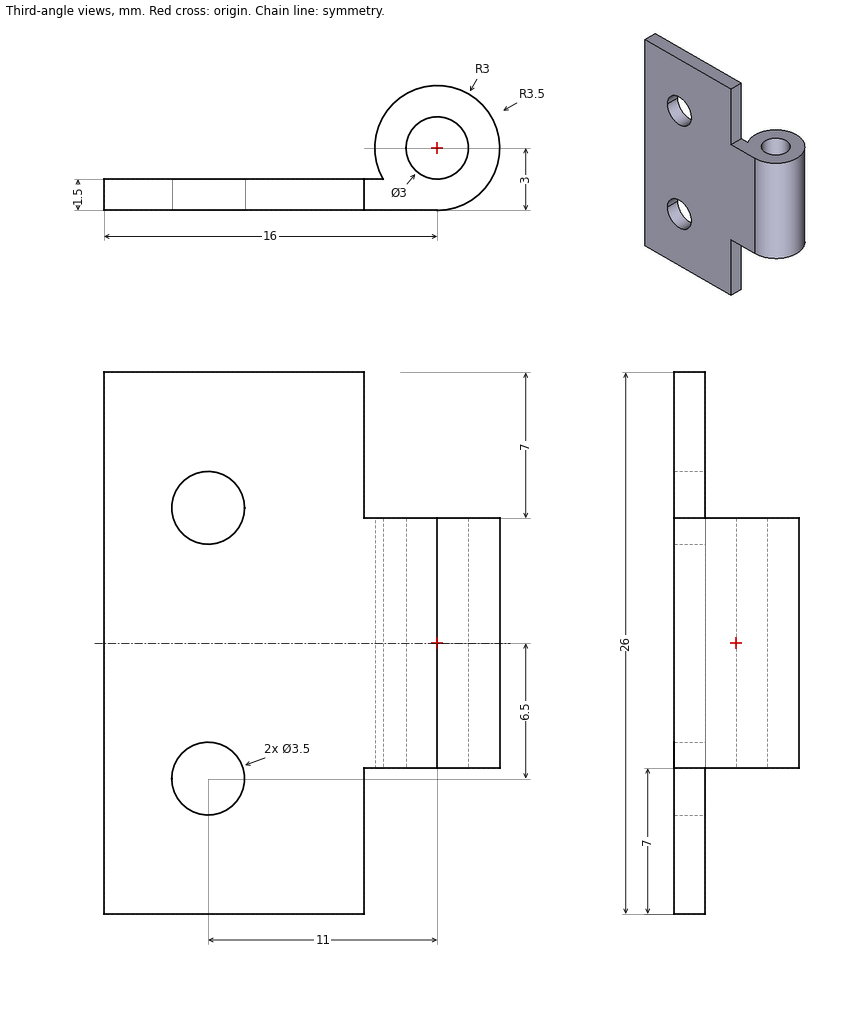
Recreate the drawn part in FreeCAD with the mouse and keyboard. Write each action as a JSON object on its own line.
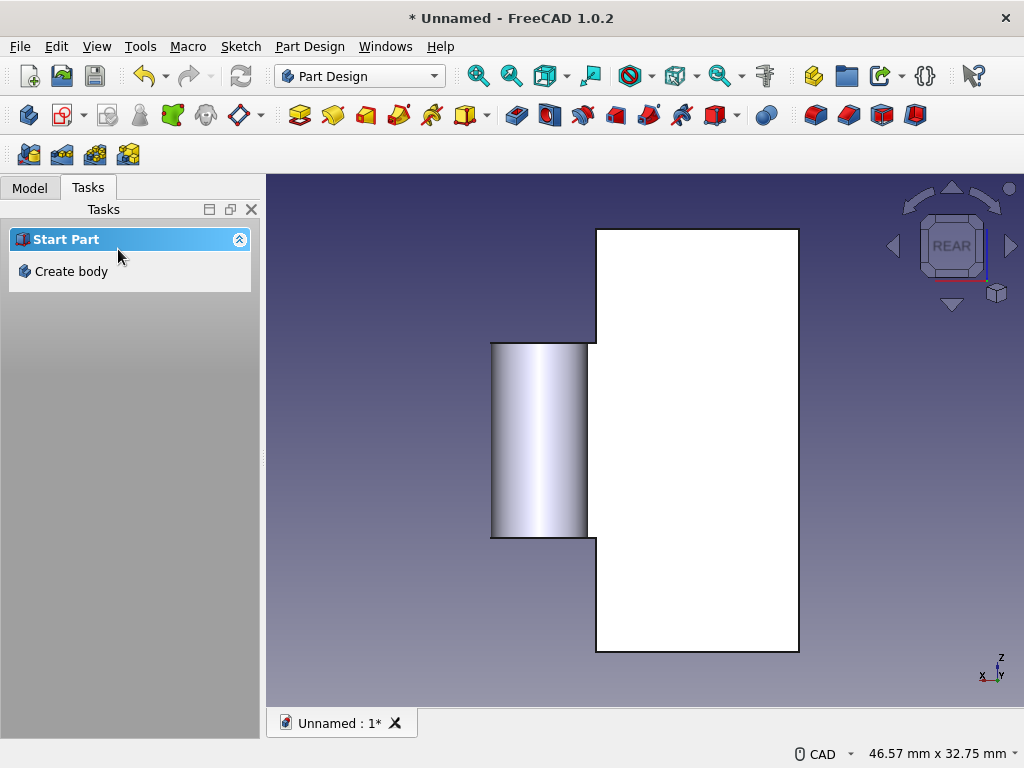
{"action": "left_click", "coordinate": [690, 439]}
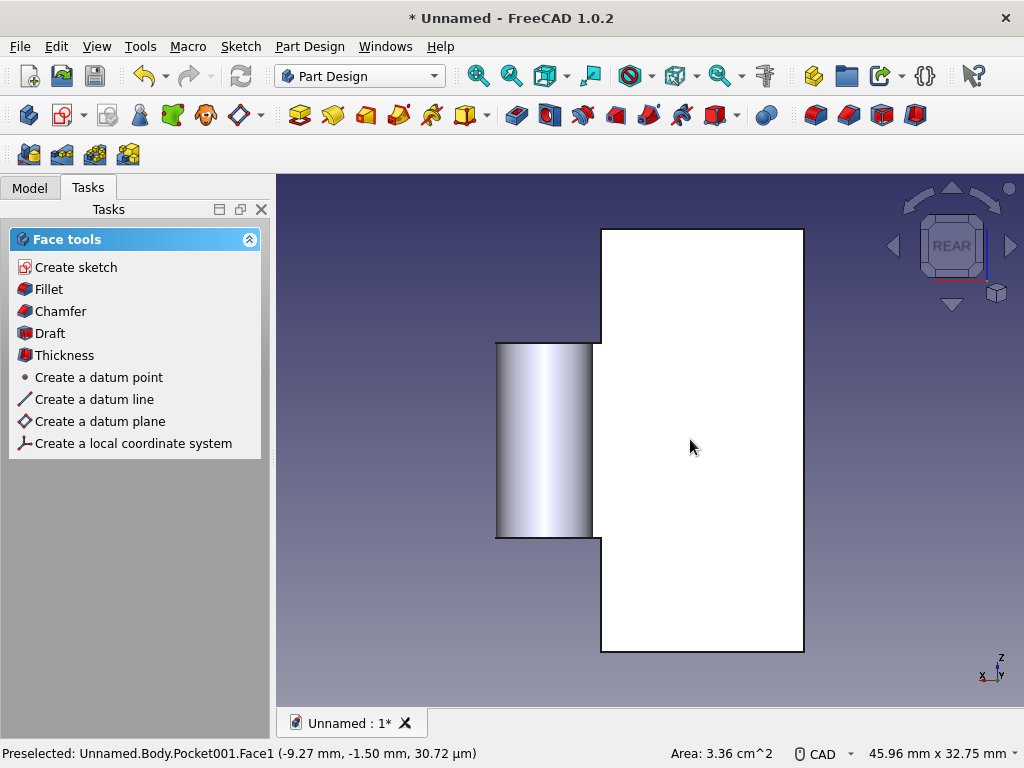
{"action": "left_click", "coordinate": [62, 116]}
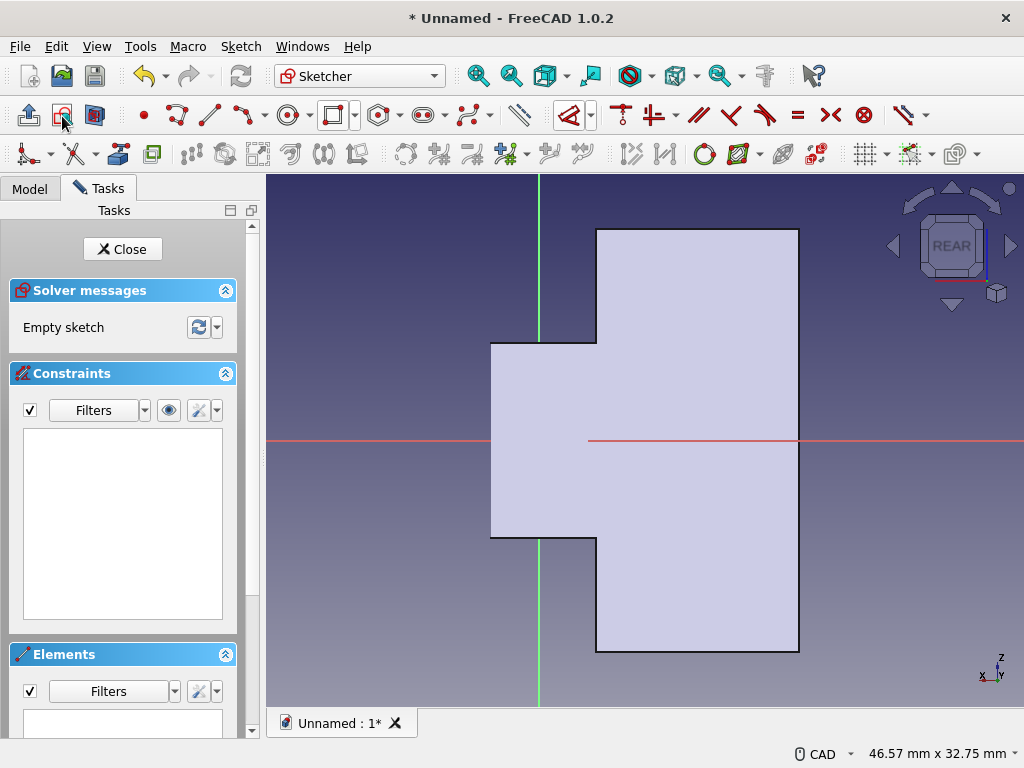
{"action": "left_click", "coordinate": [288, 116]}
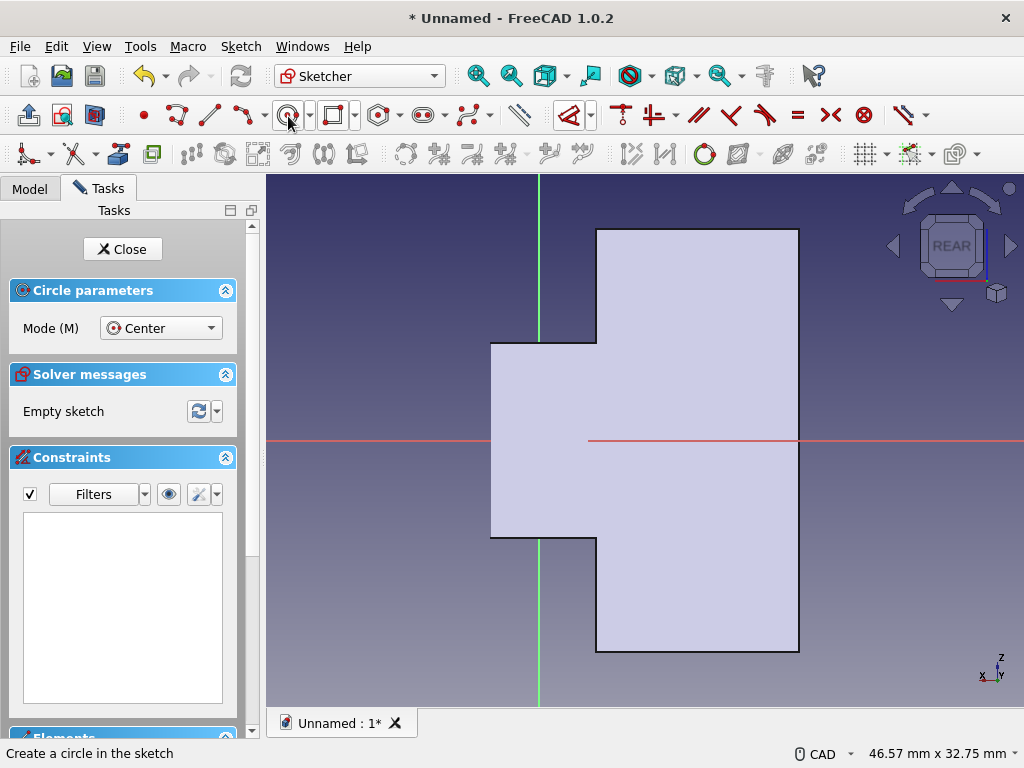
{"action": "left_click", "coordinate": [718, 546]}
{"action": "left_click", "coordinate": [738, 526]}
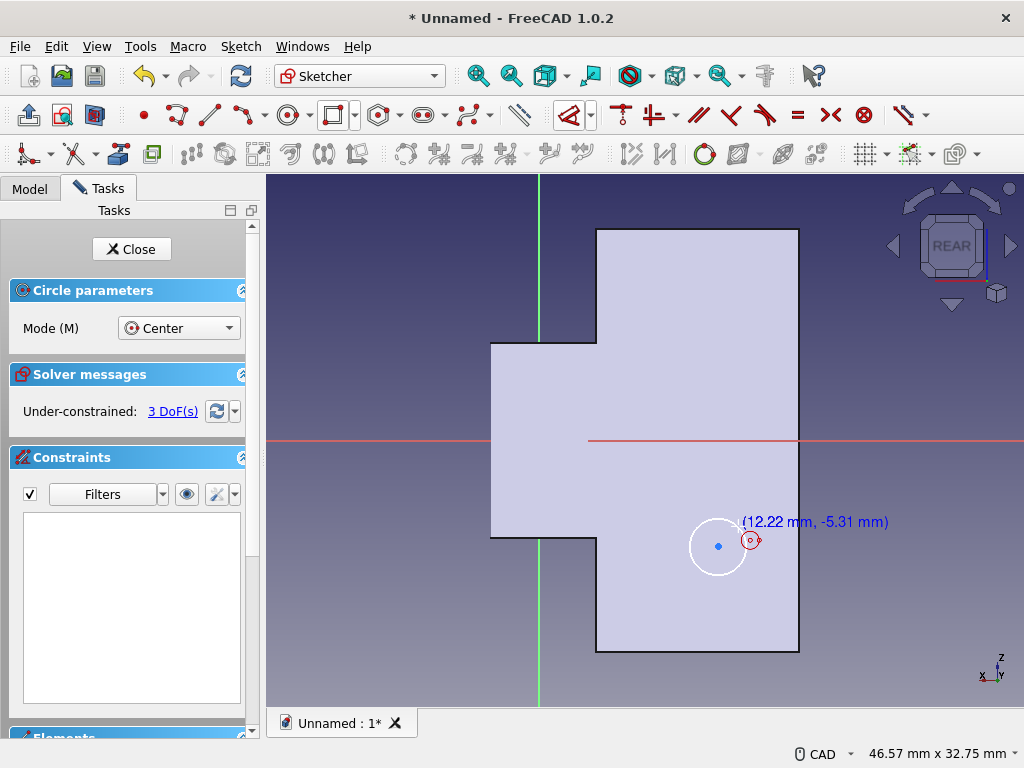
{"action": "left_click", "coordinate": [718, 335]}
{"action": "left_click", "coordinate": [738, 315]}
{"action": "key", "text": "Escape"}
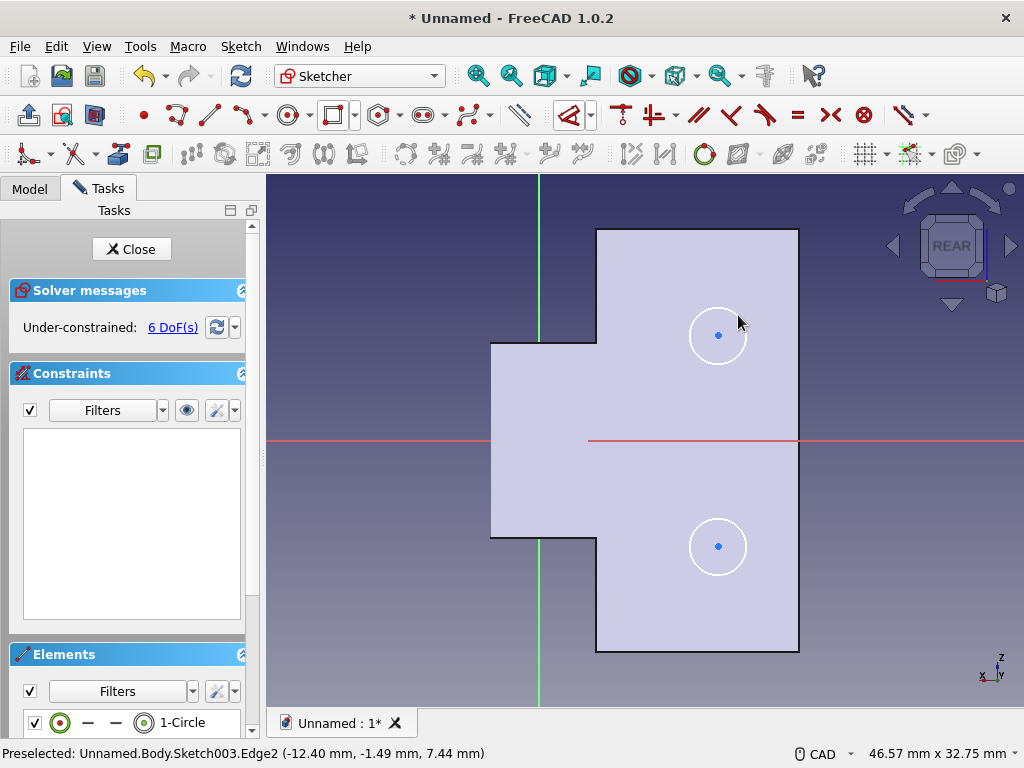
{"action": "left_click", "coordinate": [738, 527]}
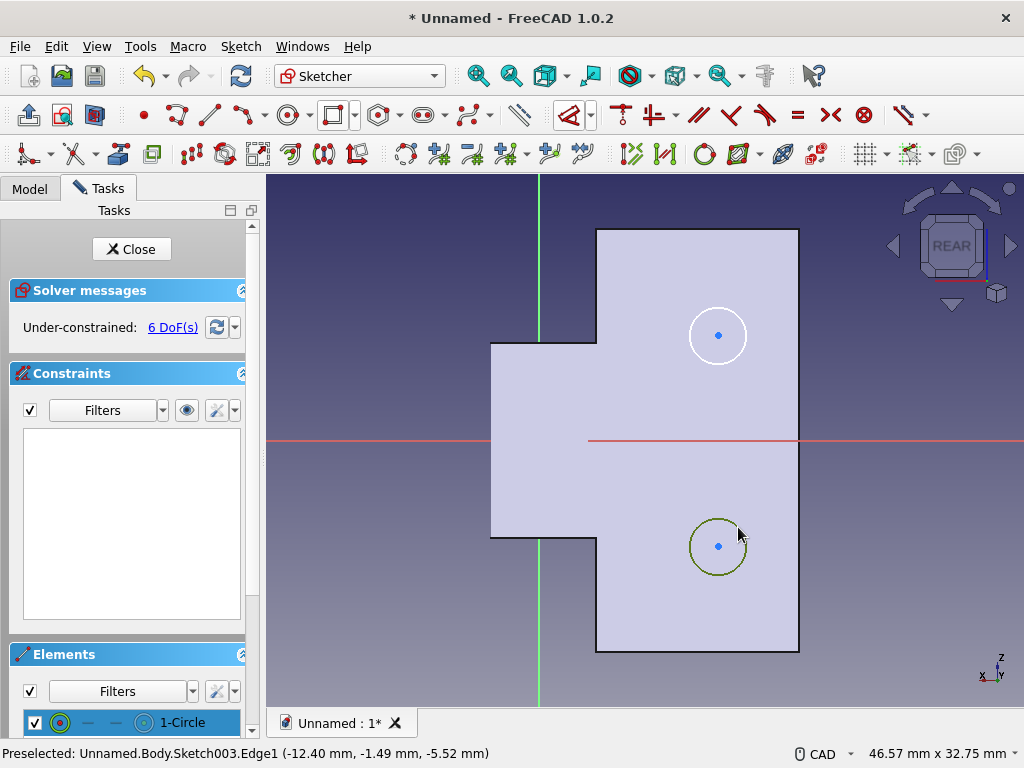
{"action": "left_click", "coordinate": [738, 316]}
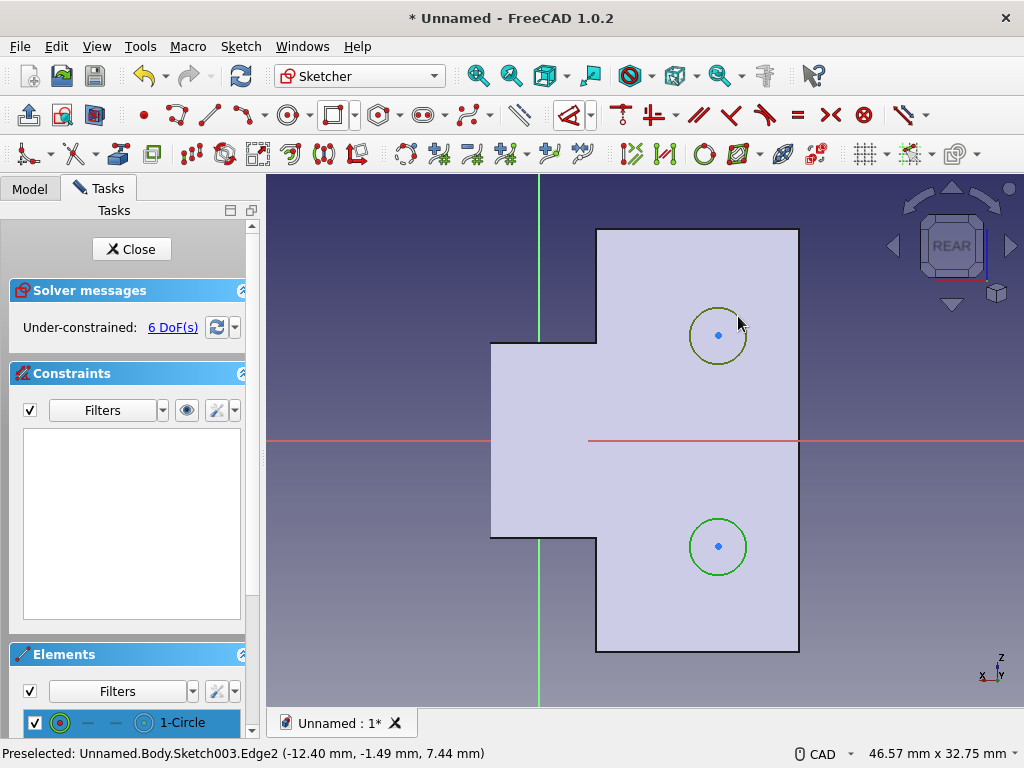
{"action": "left_click", "coordinate": [798, 116]}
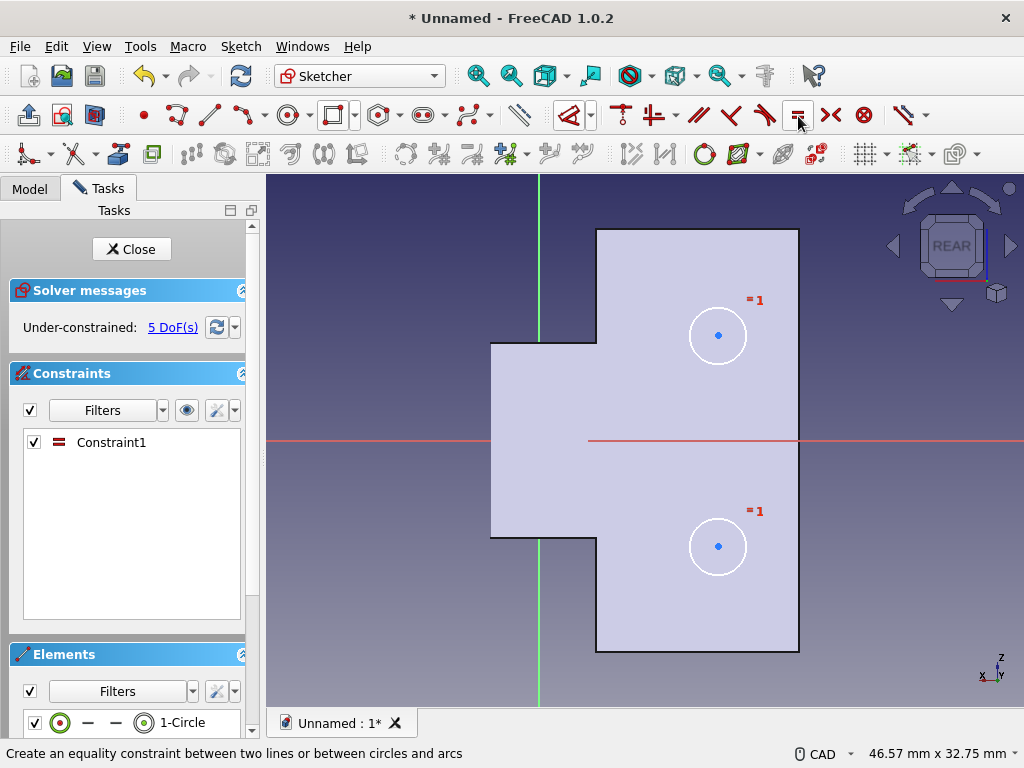
{"action": "left_click", "coordinate": [718, 547]}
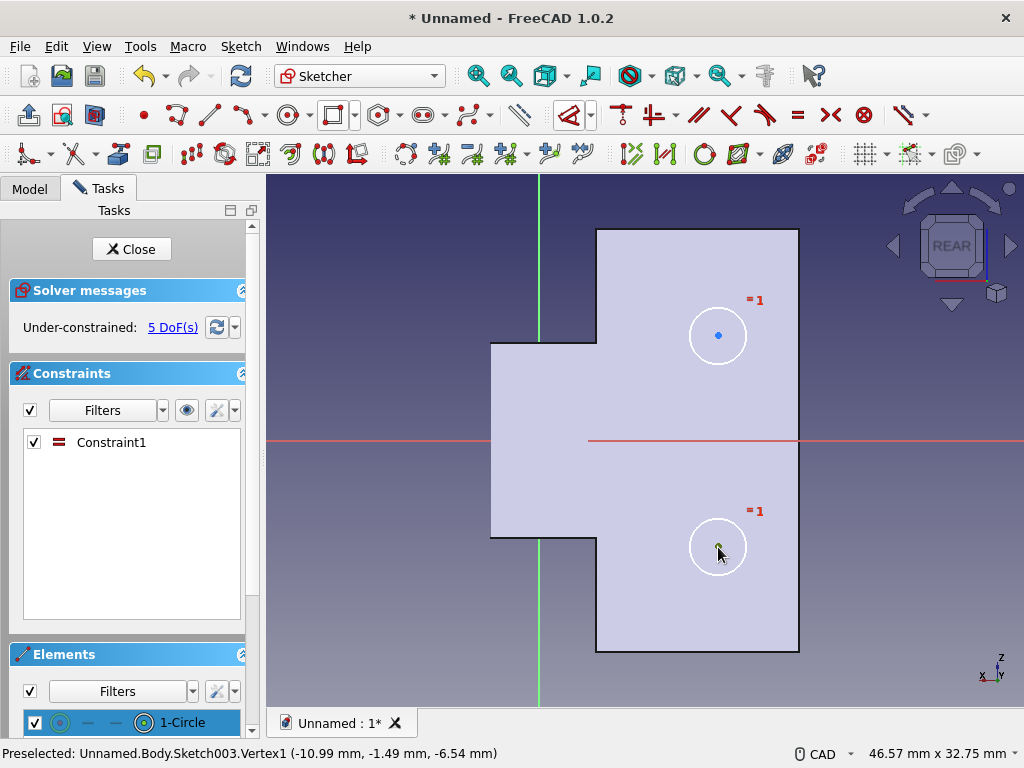
{"action": "left_click", "coordinate": [718, 336]}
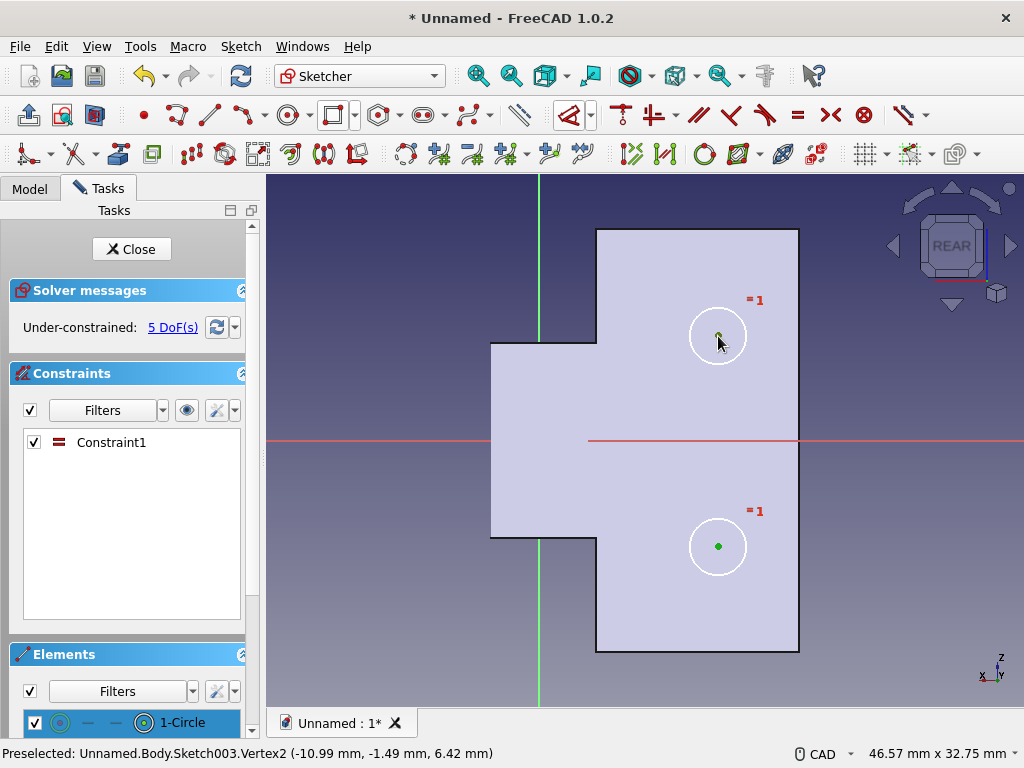
{"action": "left_click", "coordinate": [334, 440]}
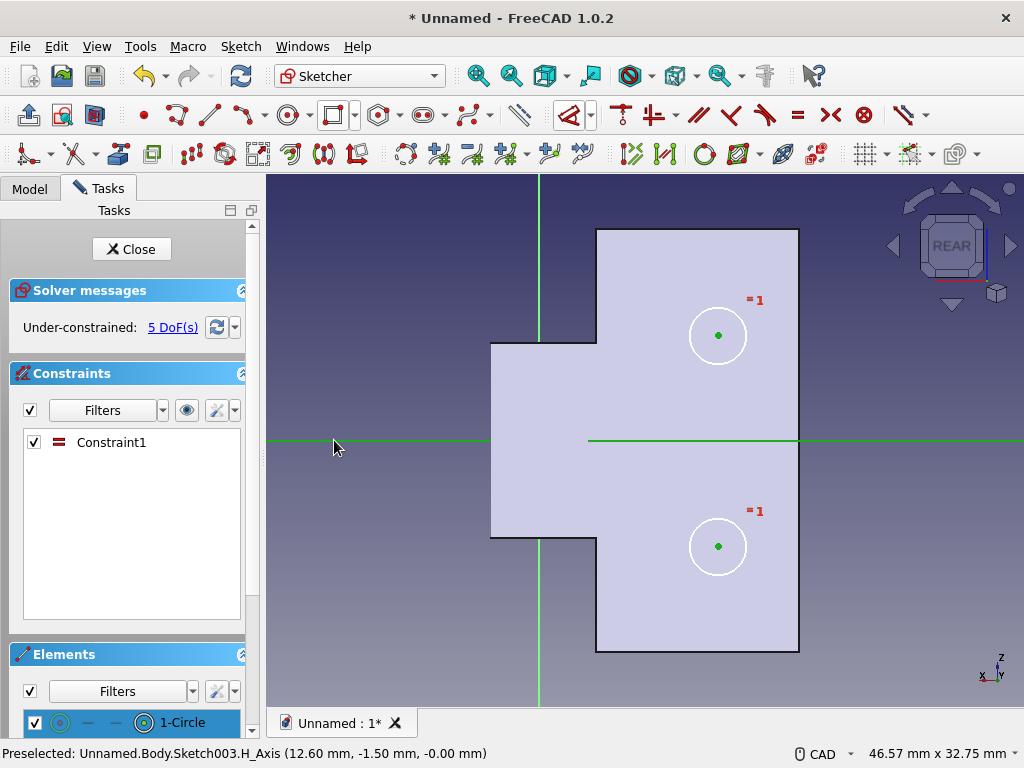
{"action": "left_click", "coordinate": [831, 116]}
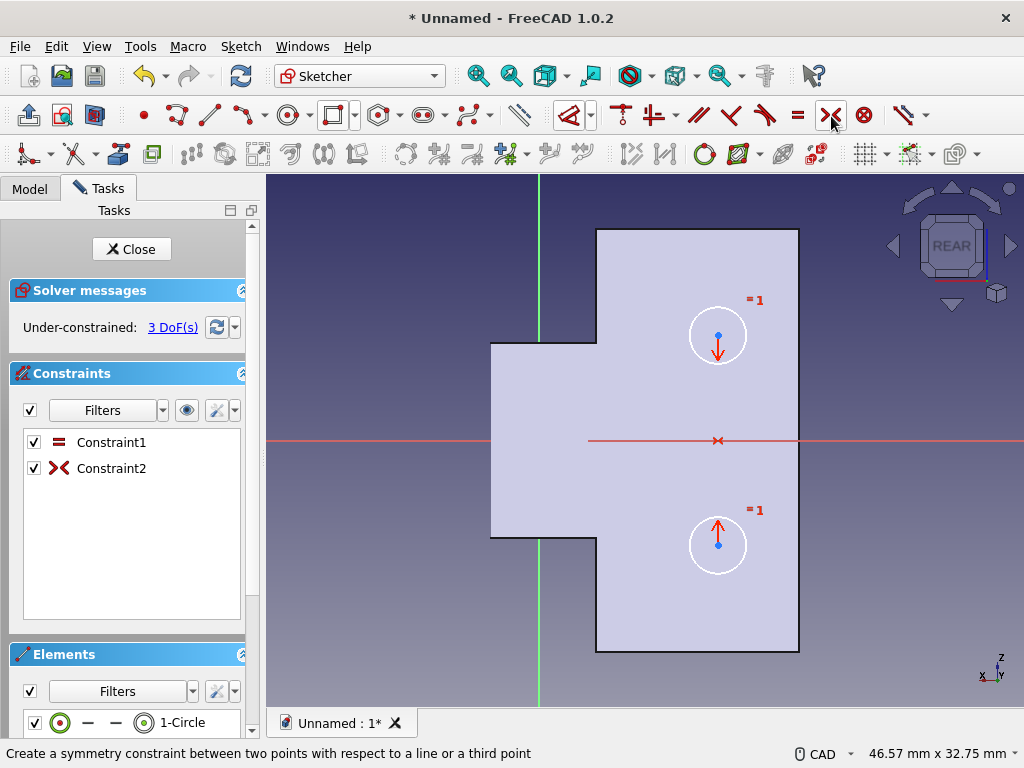
{"action": "left_click", "coordinate": [738, 525]}